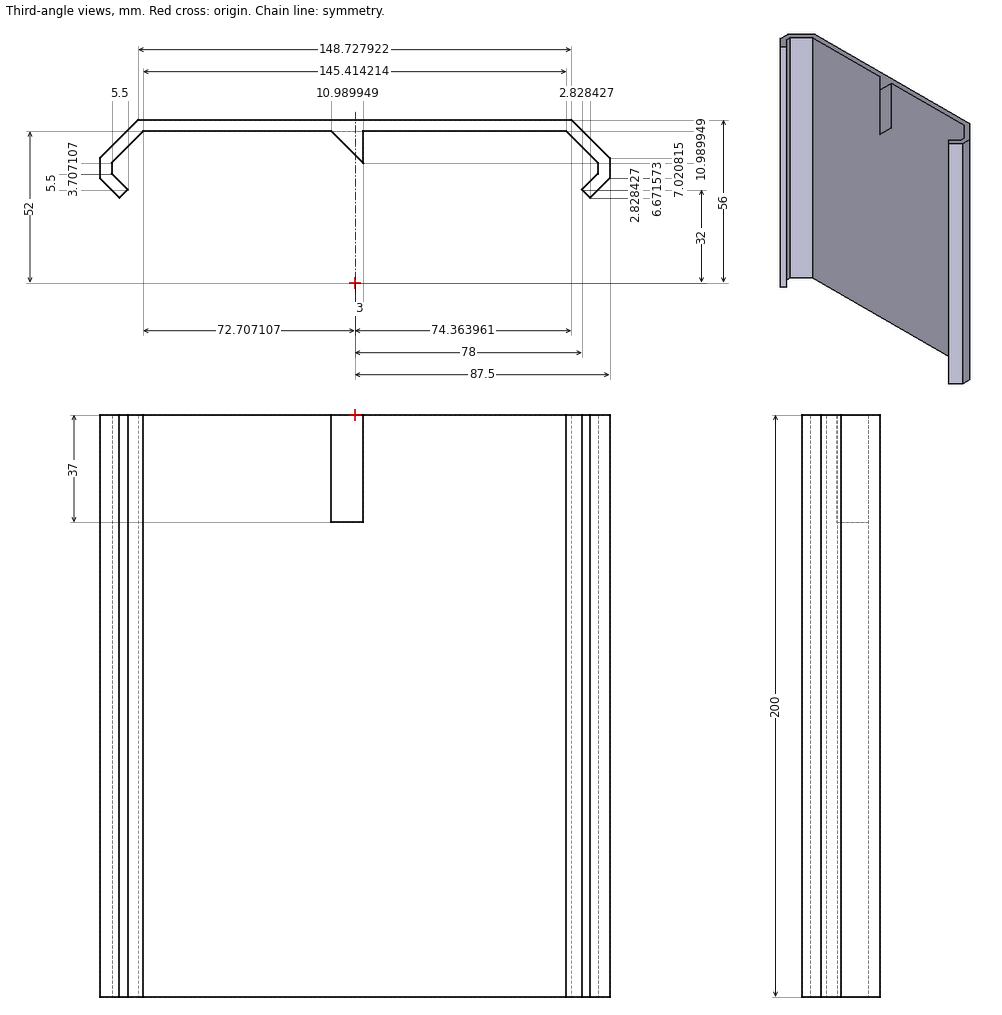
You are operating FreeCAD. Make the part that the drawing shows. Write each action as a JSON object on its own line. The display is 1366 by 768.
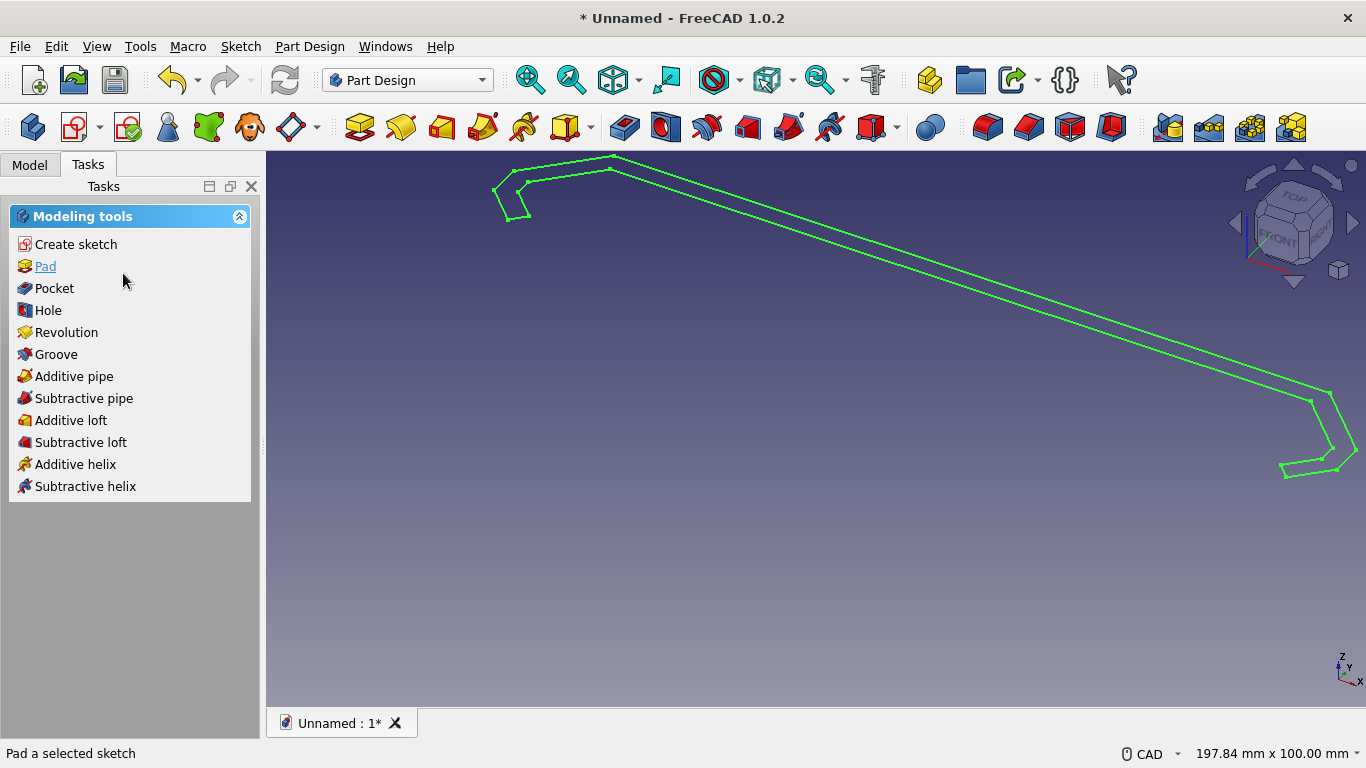
{"action": "left_click", "coordinate": [360, 128]}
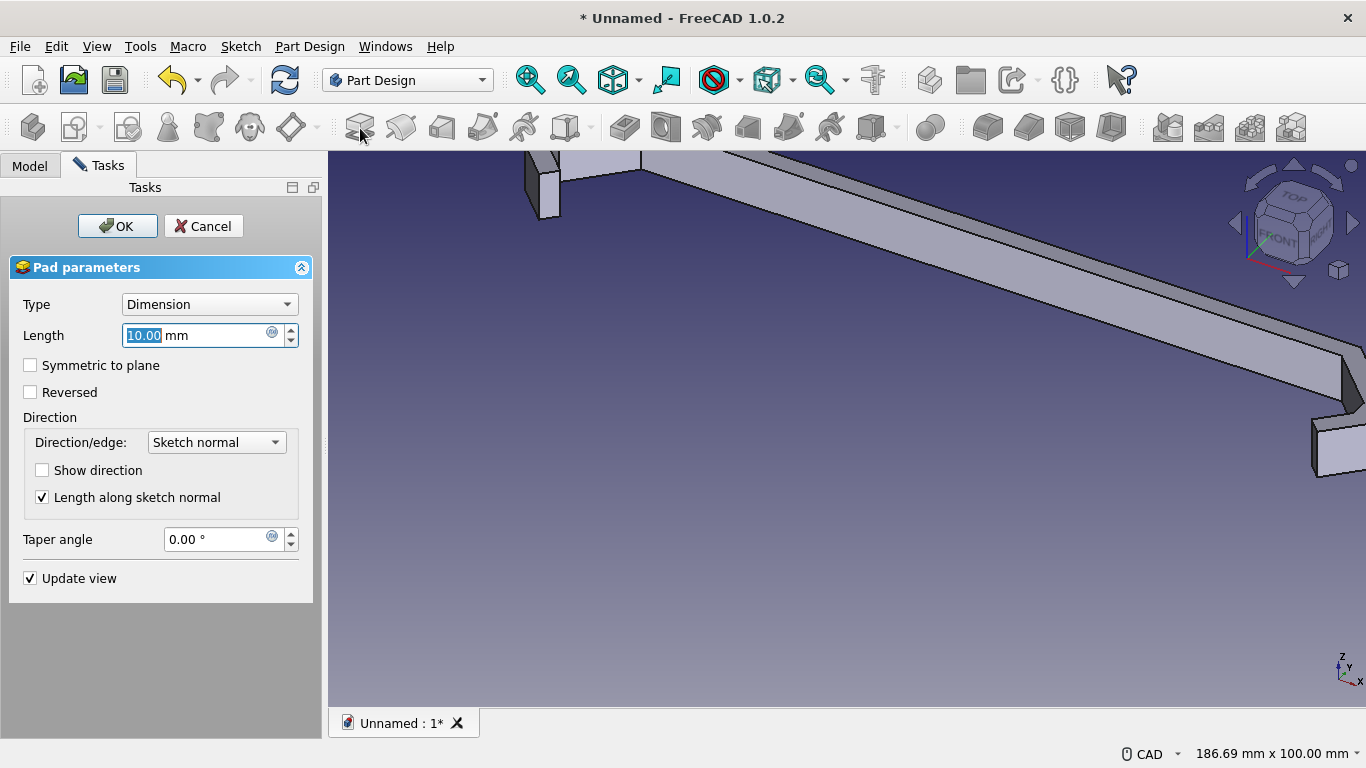
{"action": "type", "text": "200"}
{"action": "key", "text": "Tab"}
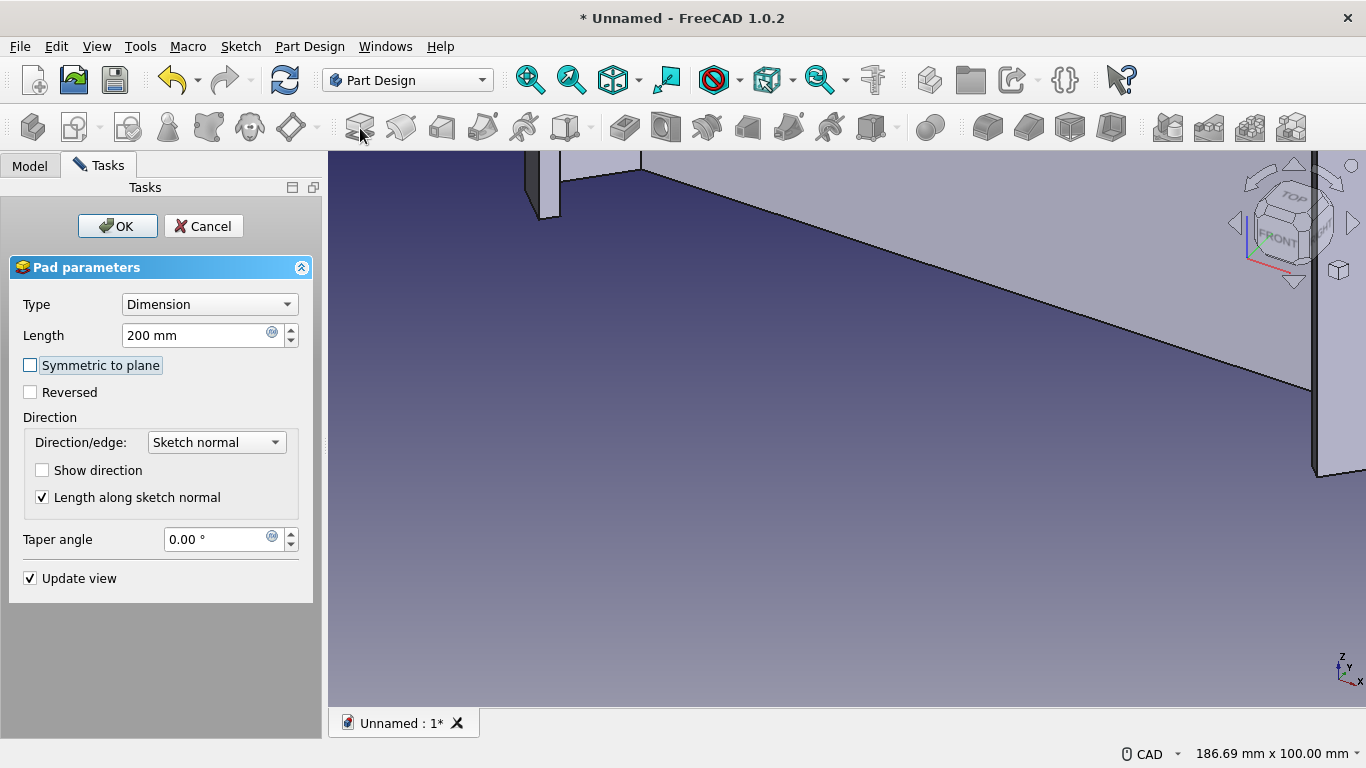
{"action": "left_click", "coordinate": [31, 392]}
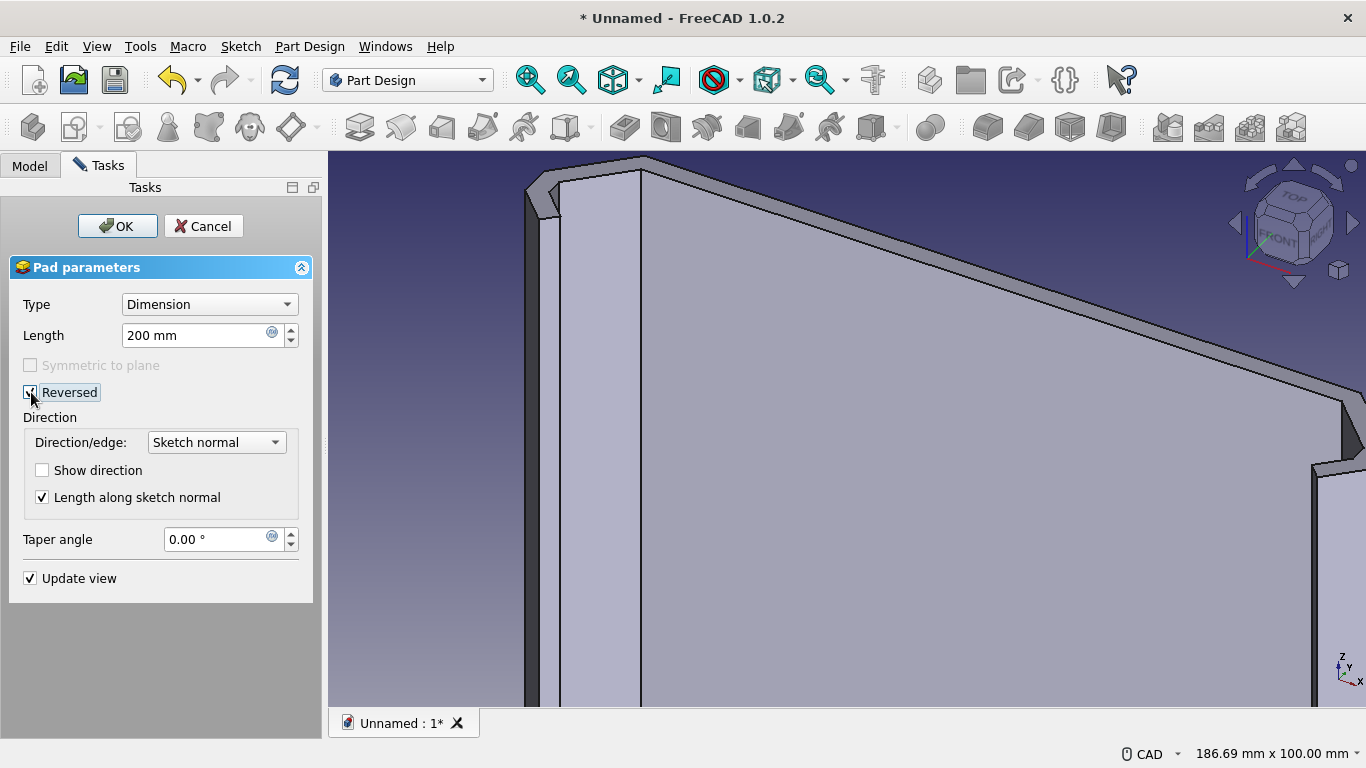
{"action": "left_click", "coordinate": [118, 226]}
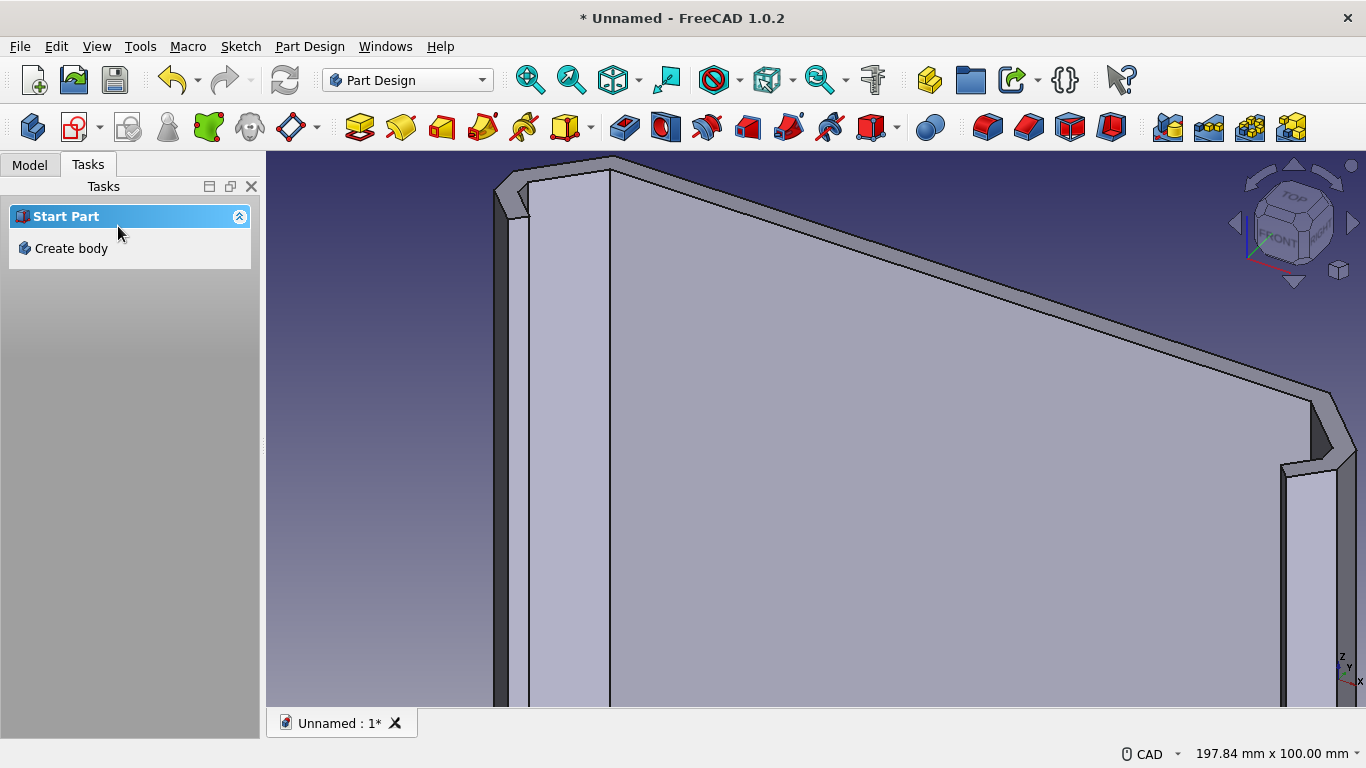
{"action": "left_click", "coordinate": [531, 80]}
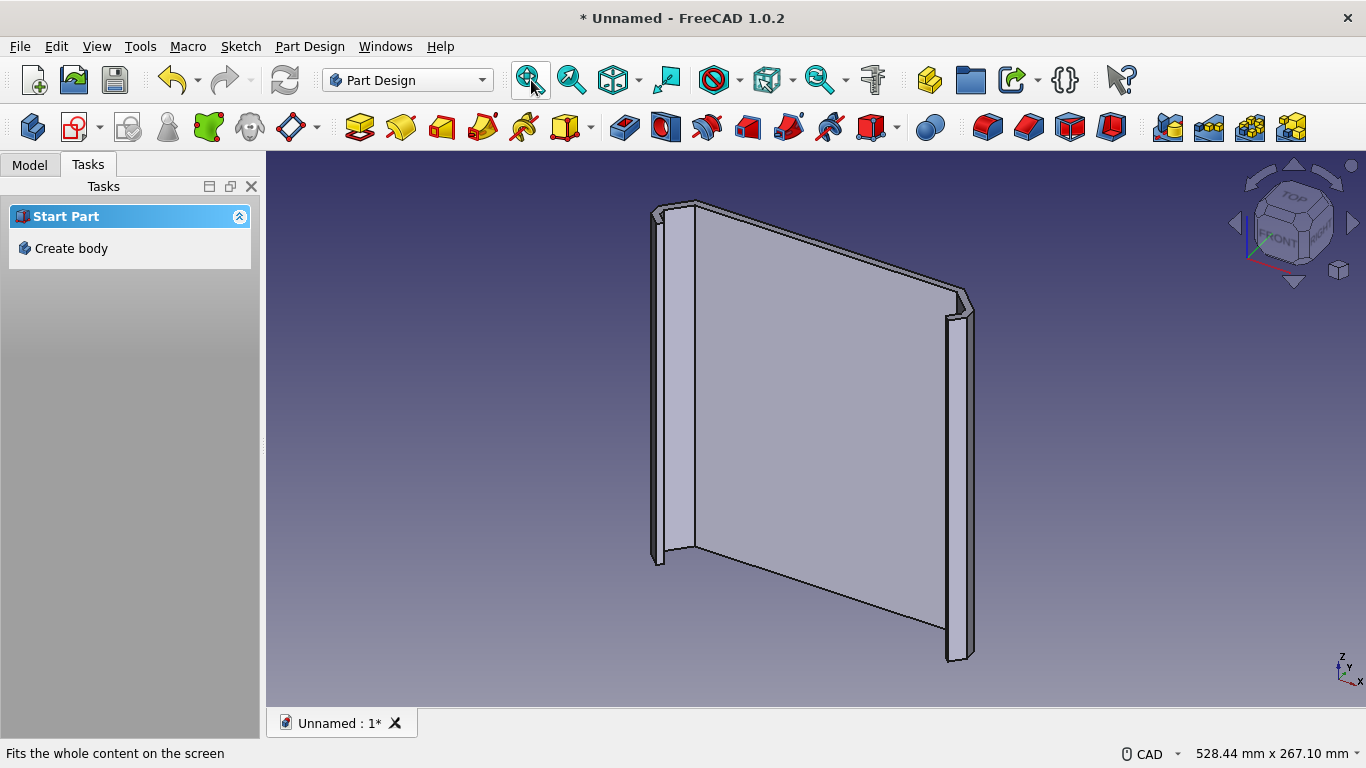
{"action": "scroll", "coordinate": [918, 275], "scroll_direction": "up", "scroll_amount": 6}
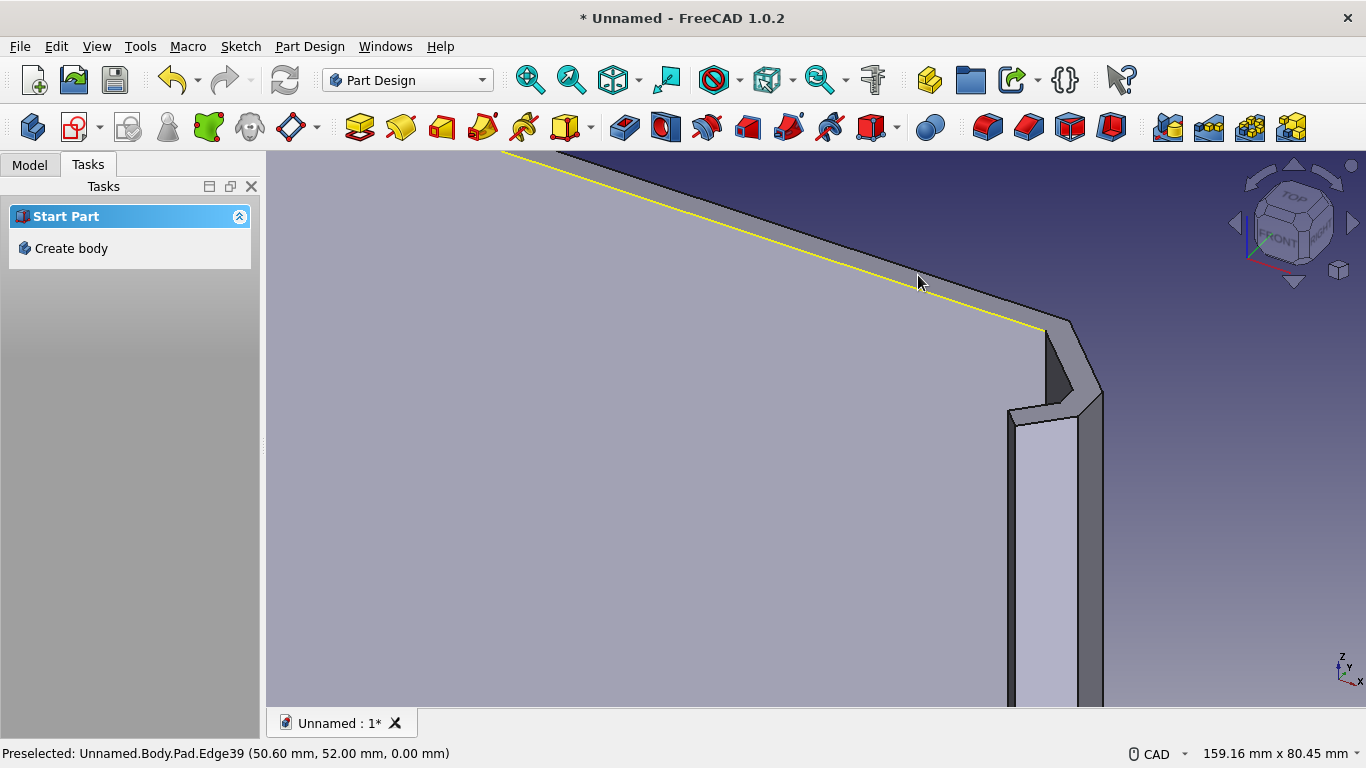
{"action": "left_click", "coordinate": [917, 278]}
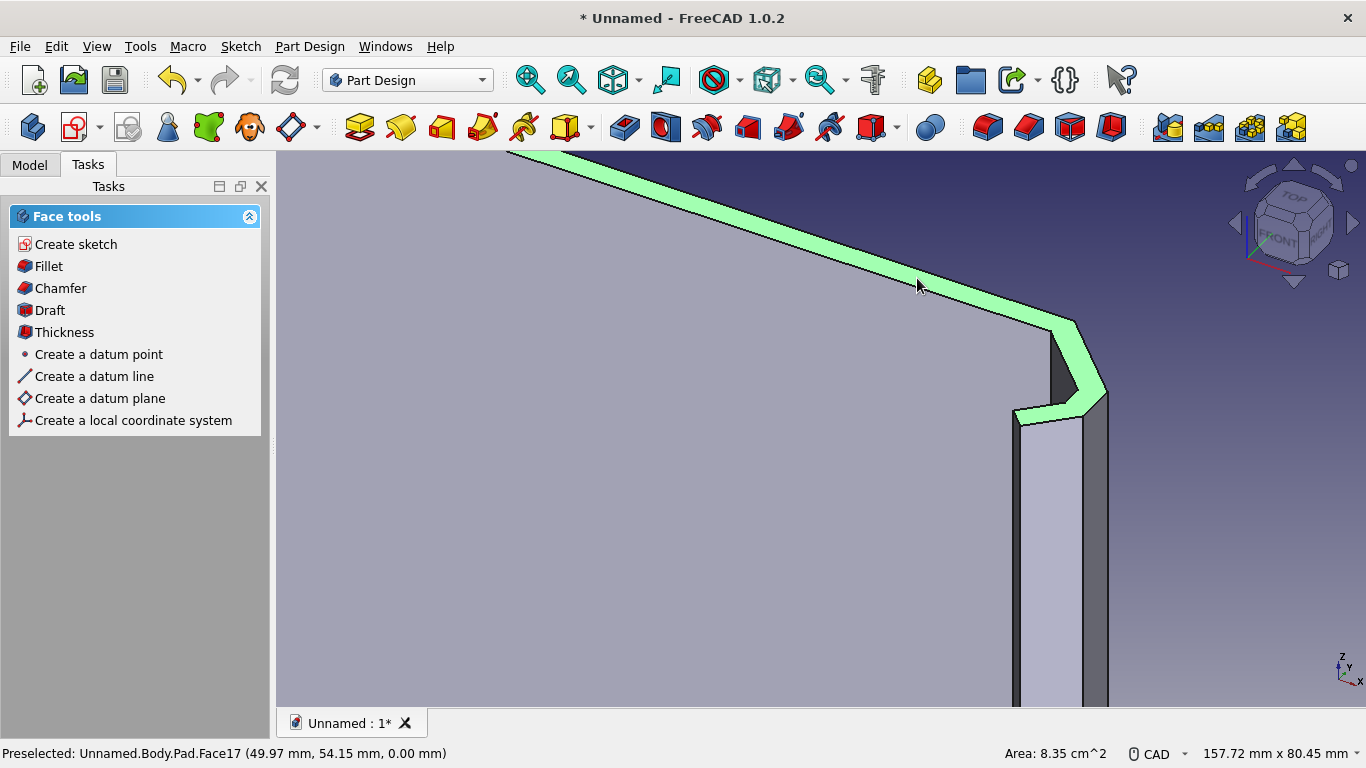
{"action": "left_click", "coordinate": [74, 128]}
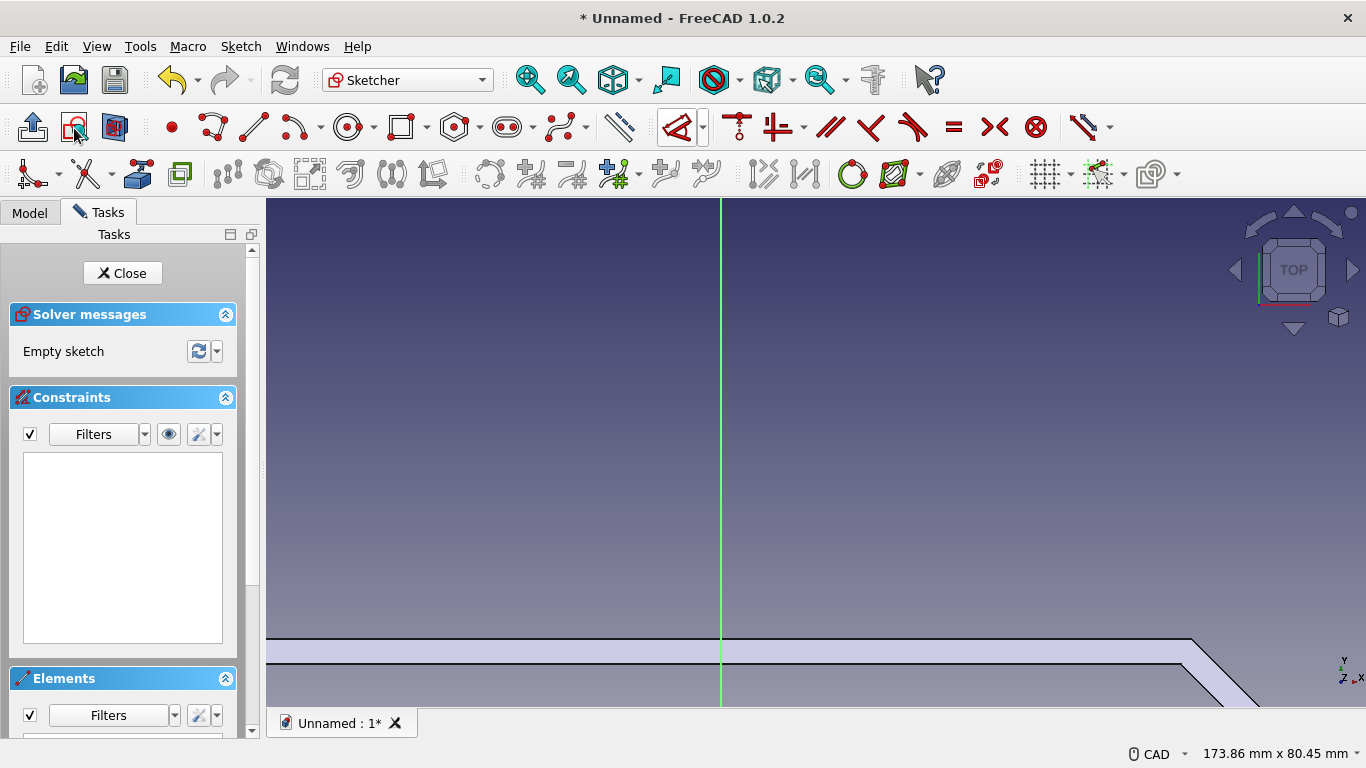
{"action": "scroll", "coordinate": [748, 452], "scroll_direction": "down", "scroll_amount": 5}